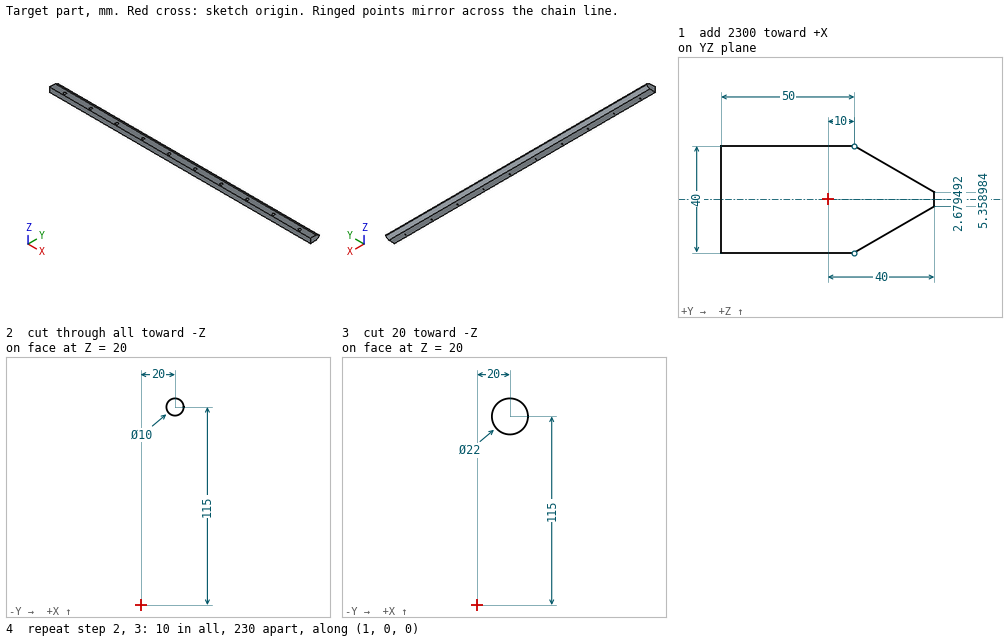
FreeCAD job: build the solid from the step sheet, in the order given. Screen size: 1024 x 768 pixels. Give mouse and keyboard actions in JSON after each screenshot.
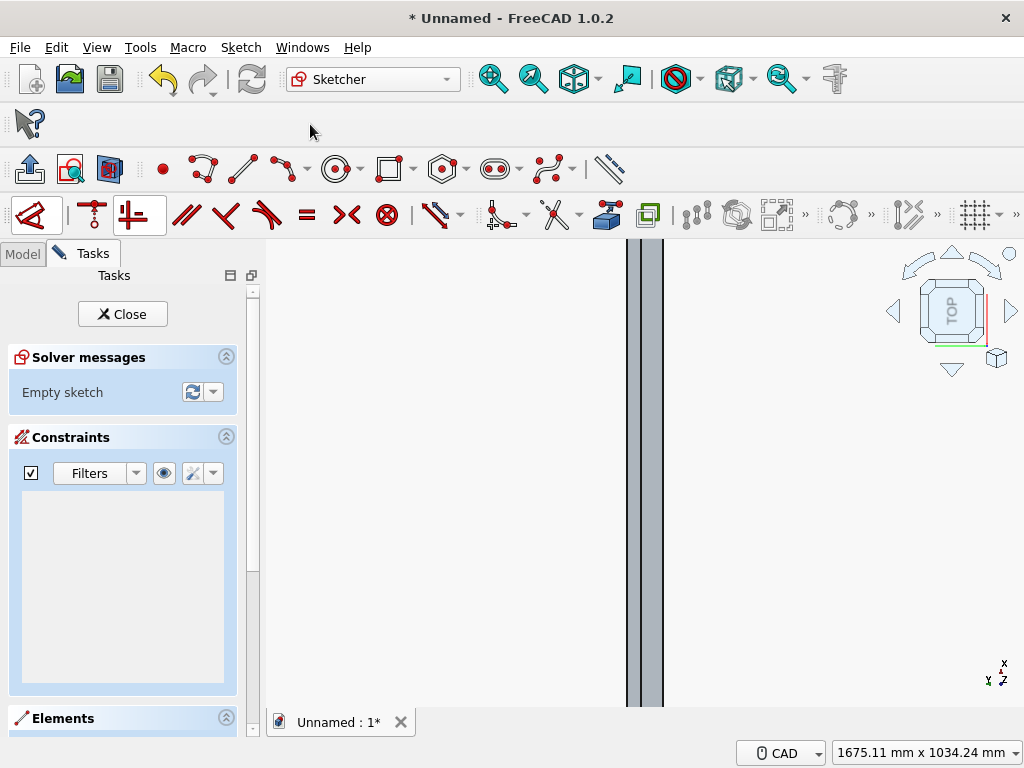
{"action": "scroll", "coordinate": [576, 473], "scroll_direction": "down", "scroll_amount": 5}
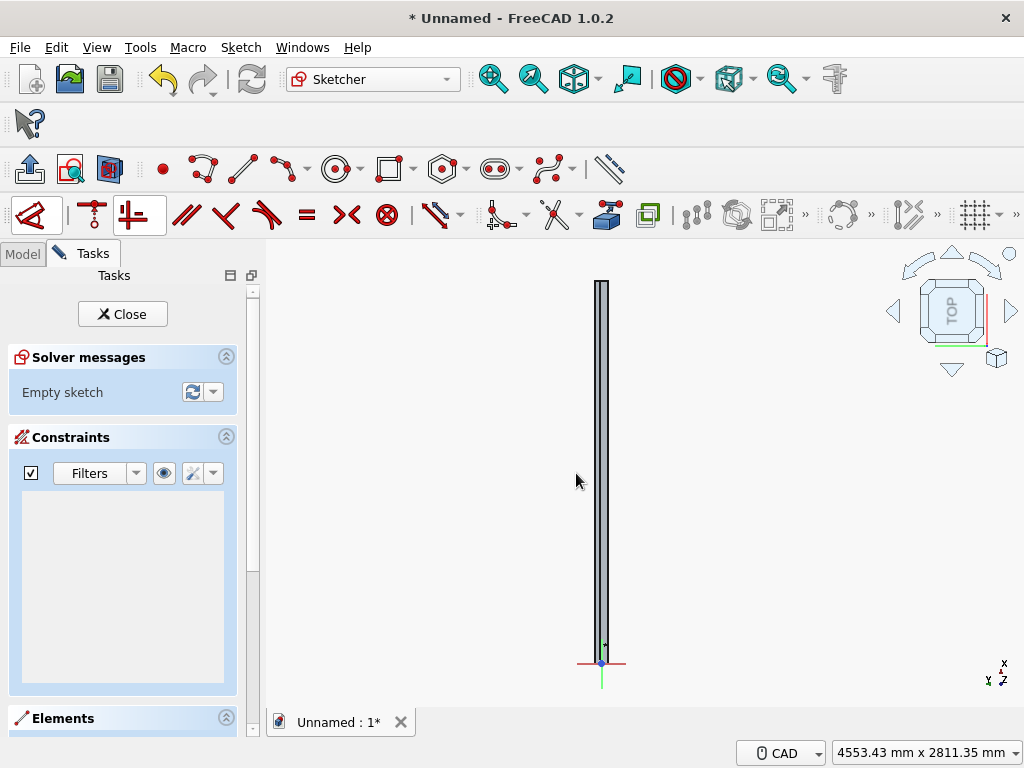
{"action": "scroll", "coordinate": [607, 654], "scroll_direction": "up", "scroll_amount": 15}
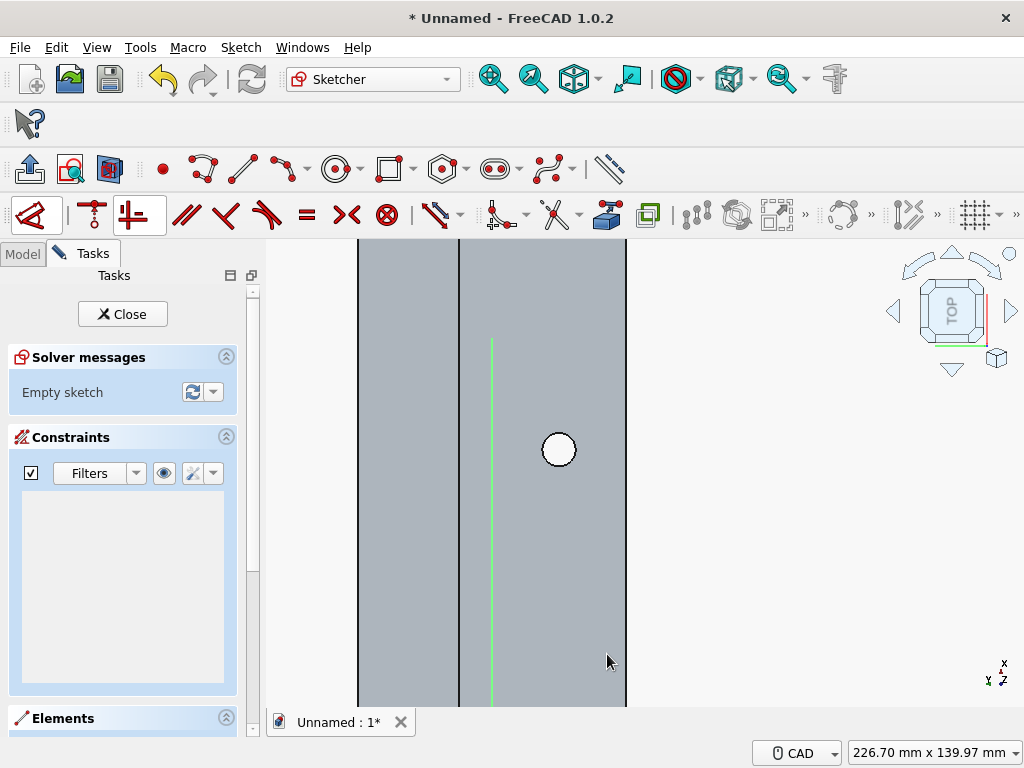
{"action": "scroll", "coordinate": [553, 442], "scroll_direction": "up", "scroll_amount": 7}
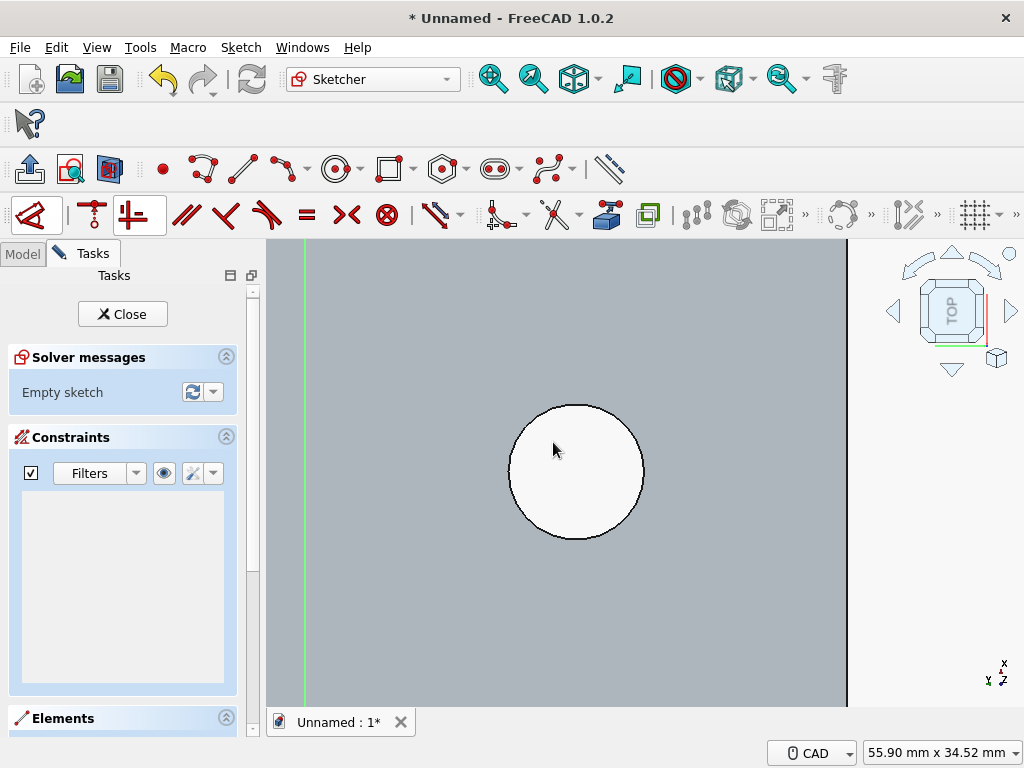
{"action": "key", "text": "g c"}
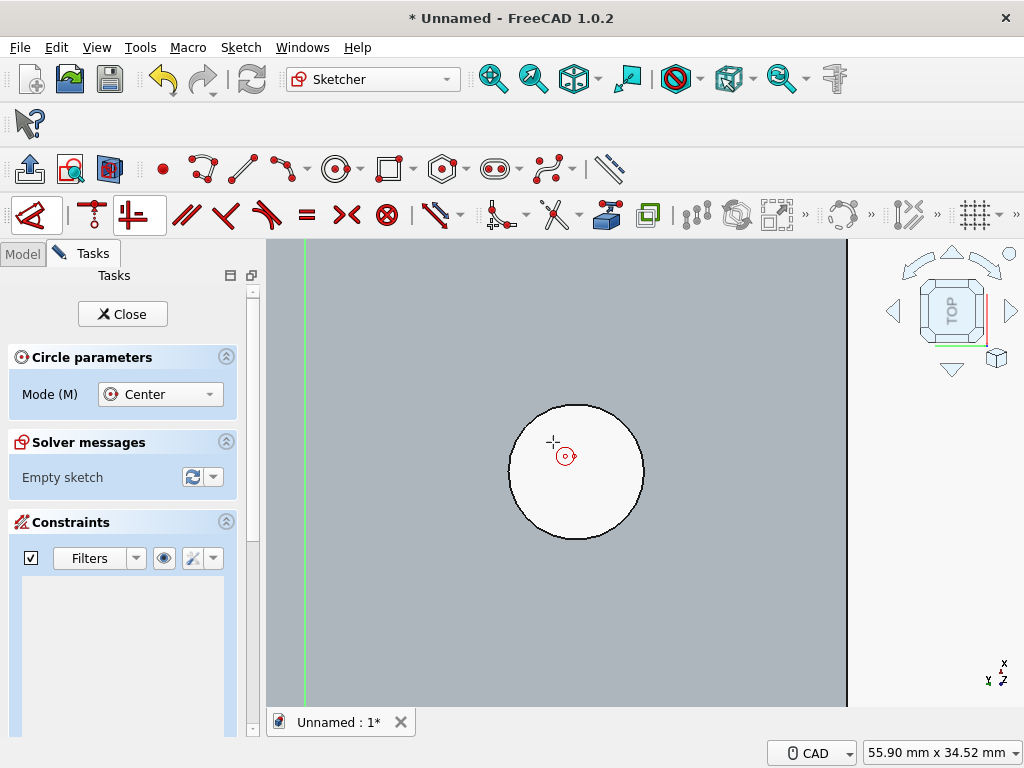
{"action": "left_click", "coordinate": [576, 472]}
{"action": "mouse_move", "coordinate": [682, 366]}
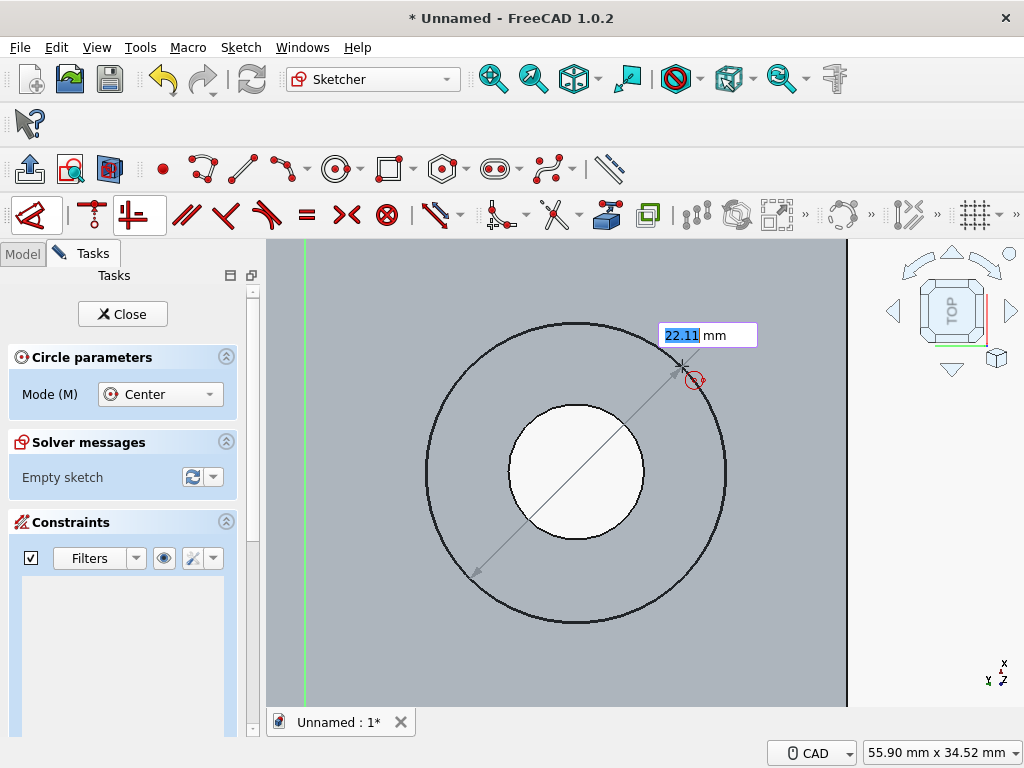
{"action": "type", "text": "22"}
{"action": "key", "text": "Return"}
{"action": "key", "text": "Escape"}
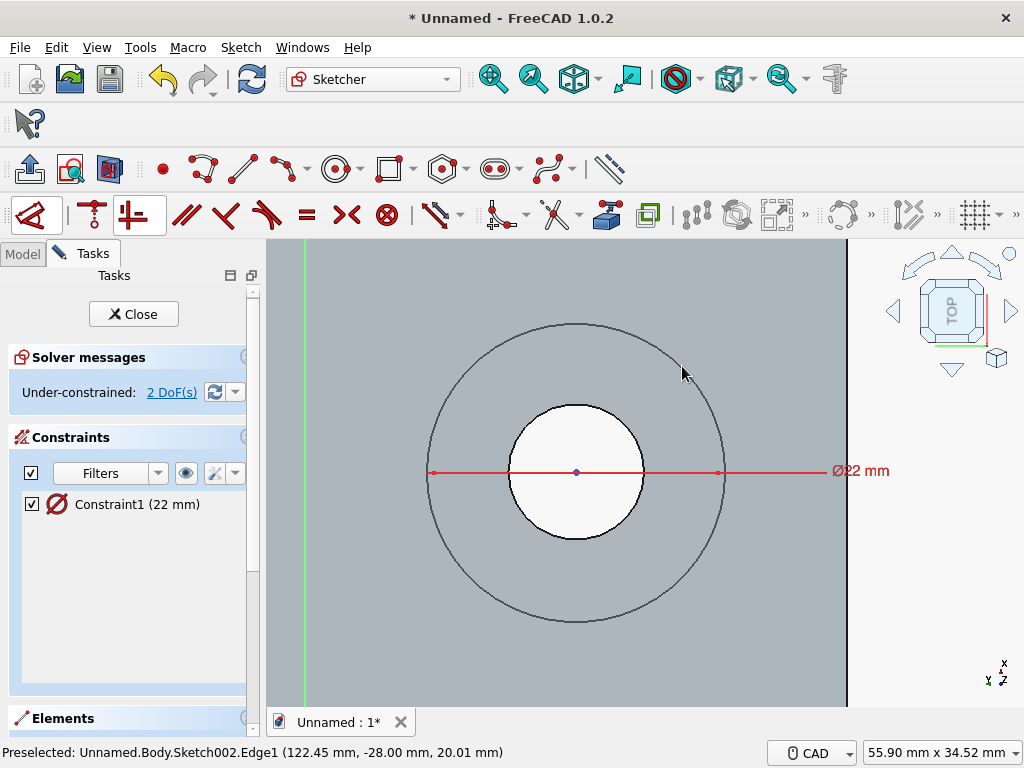
{"action": "left_click", "coordinate": [576, 473]}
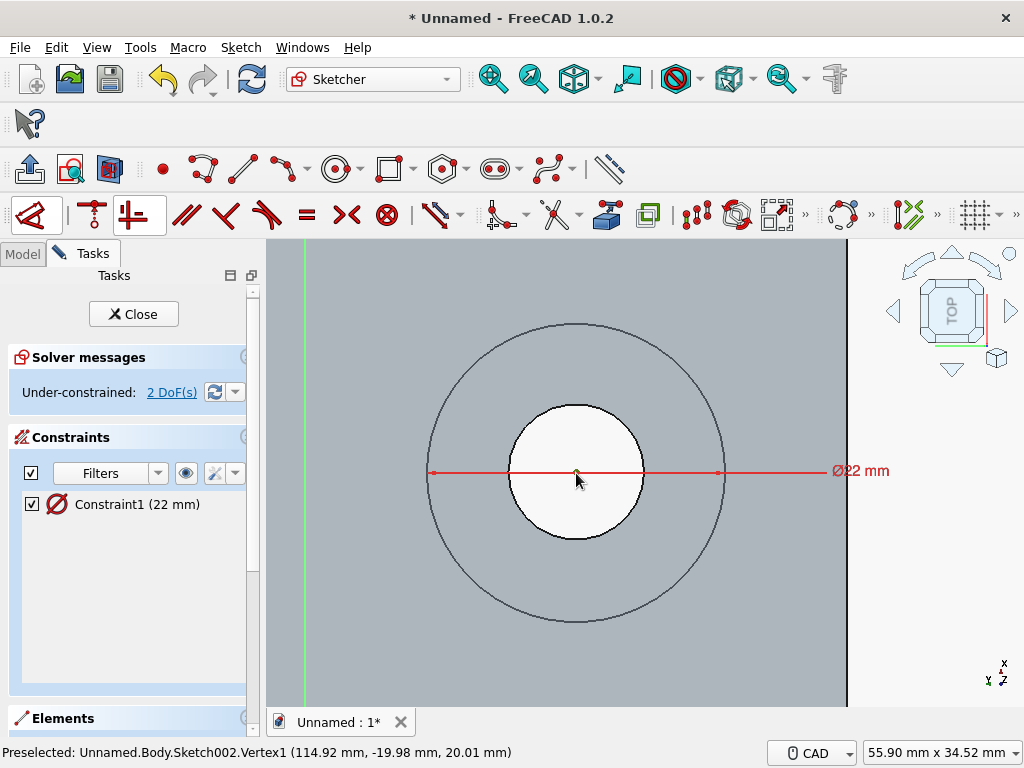
{"action": "key", "text": "l"}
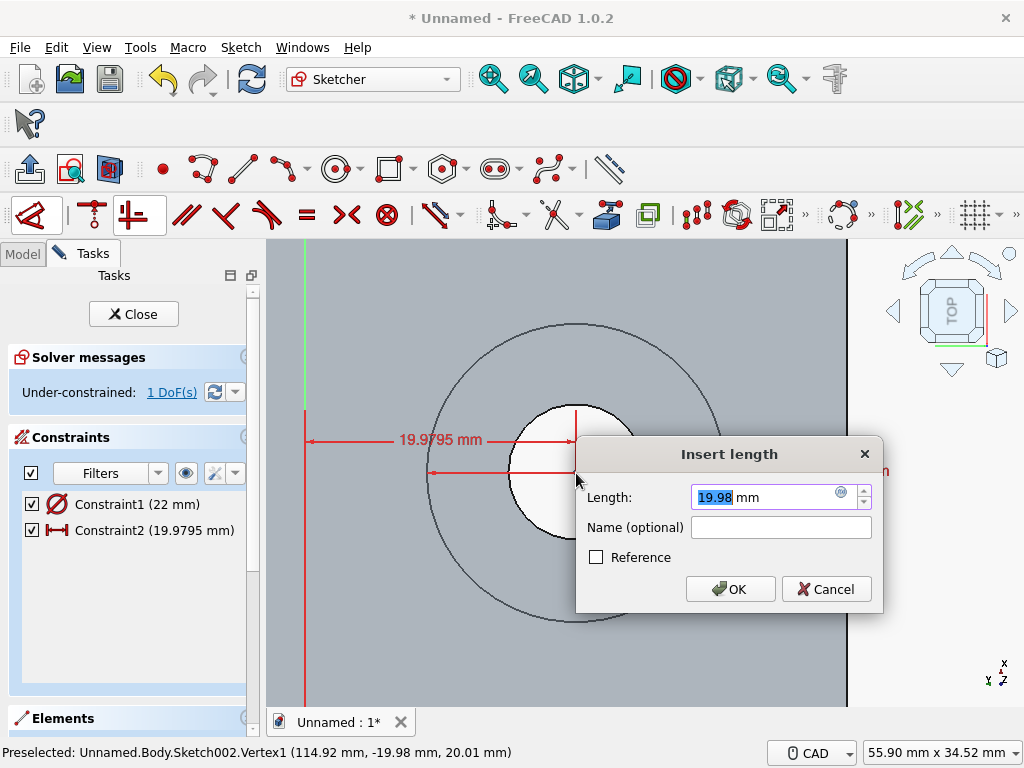
{"action": "type", "text": "20"}
{"action": "key", "text": "Return"}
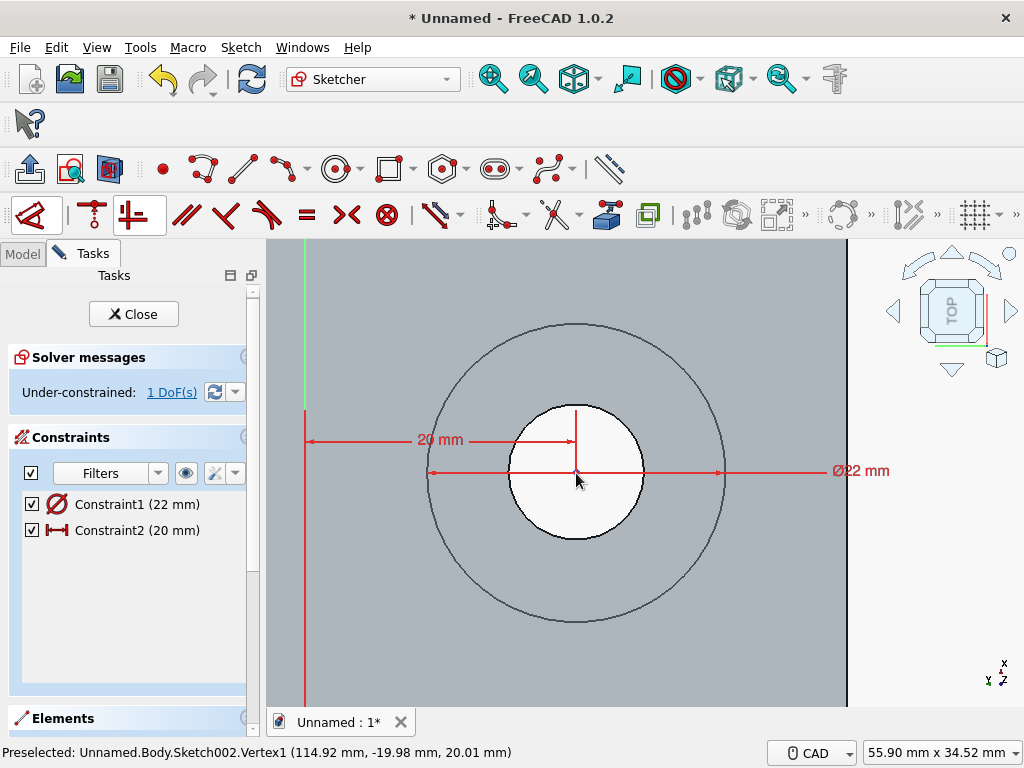
{"action": "left_click", "coordinate": [576, 473]}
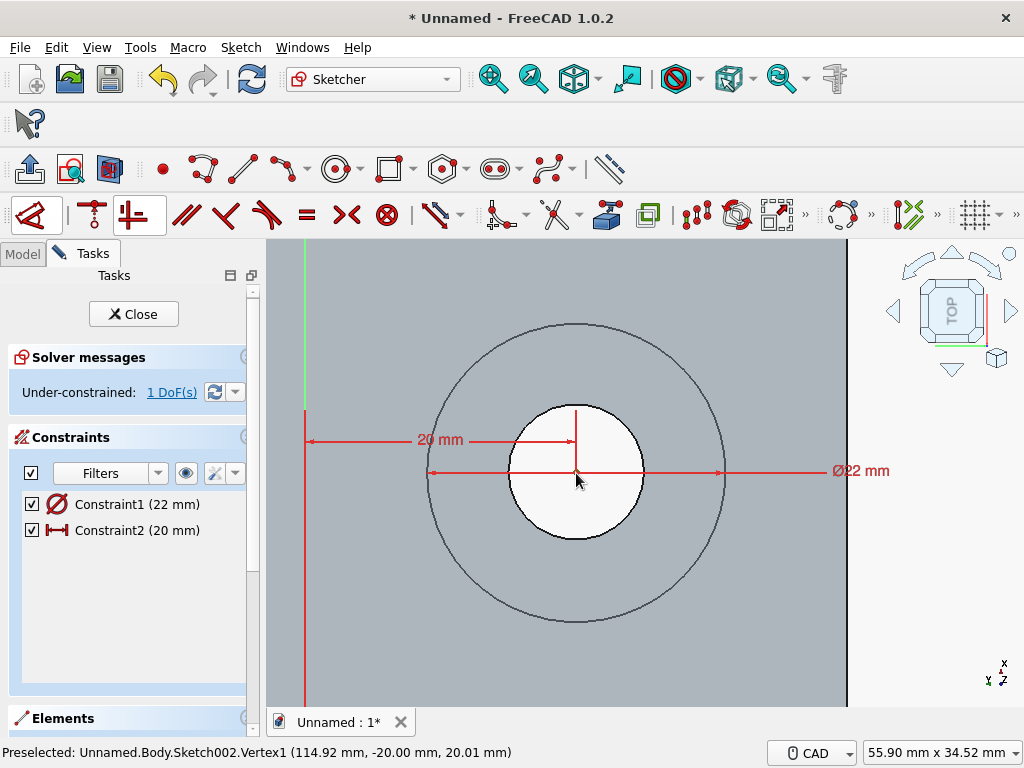
{"action": "key", "text": "i"}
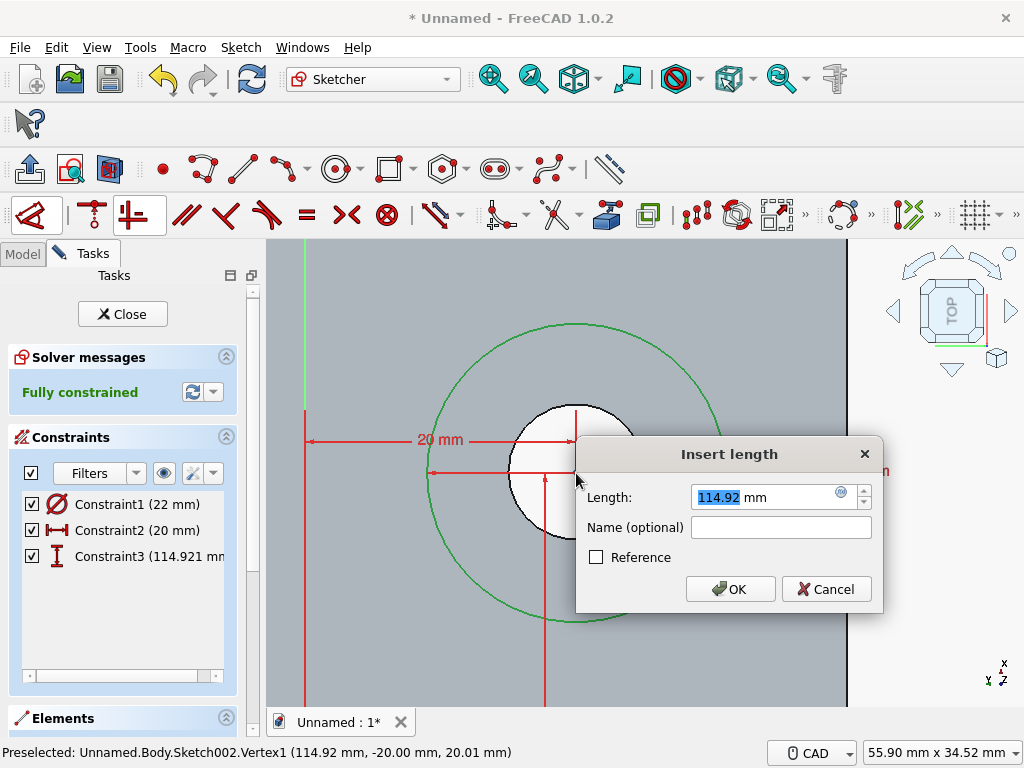
{"action": "type", "text": "115"}
{"action": "key", "text": "Return"}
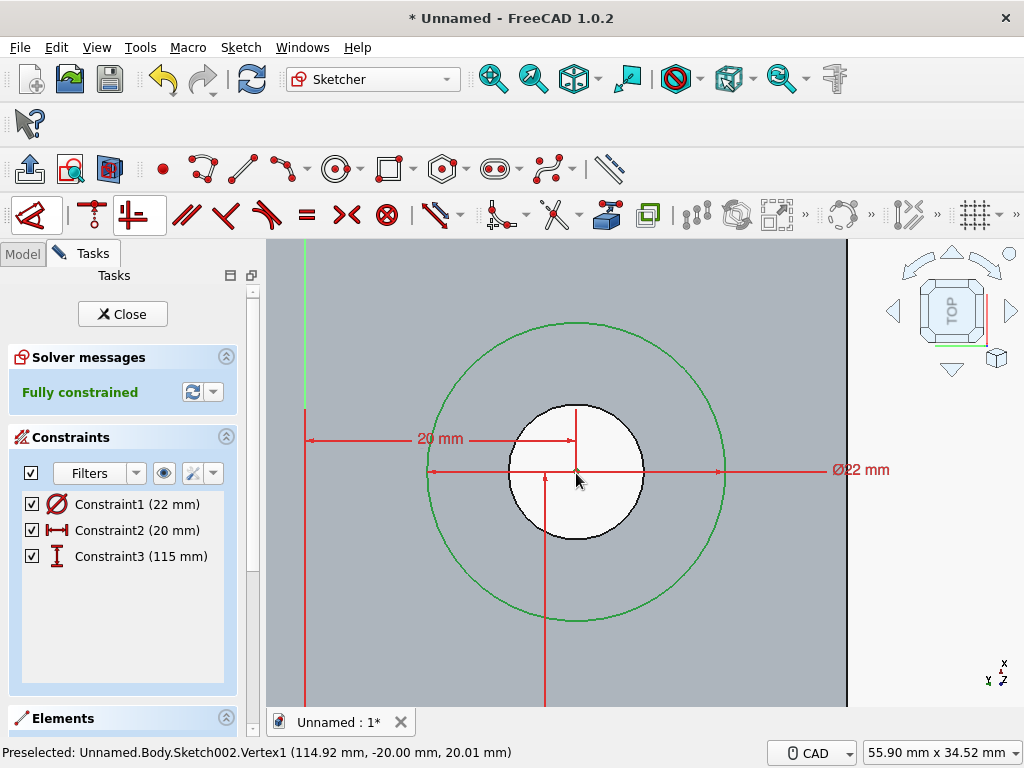
{"action": "left_click", "coordinate": [123, 314]}